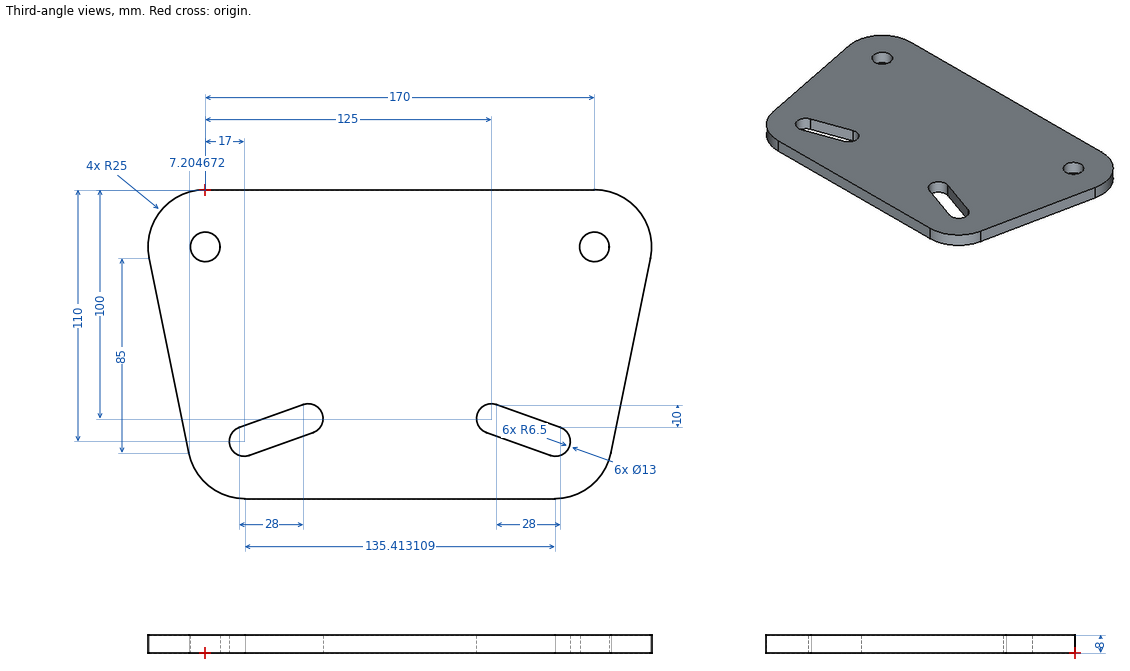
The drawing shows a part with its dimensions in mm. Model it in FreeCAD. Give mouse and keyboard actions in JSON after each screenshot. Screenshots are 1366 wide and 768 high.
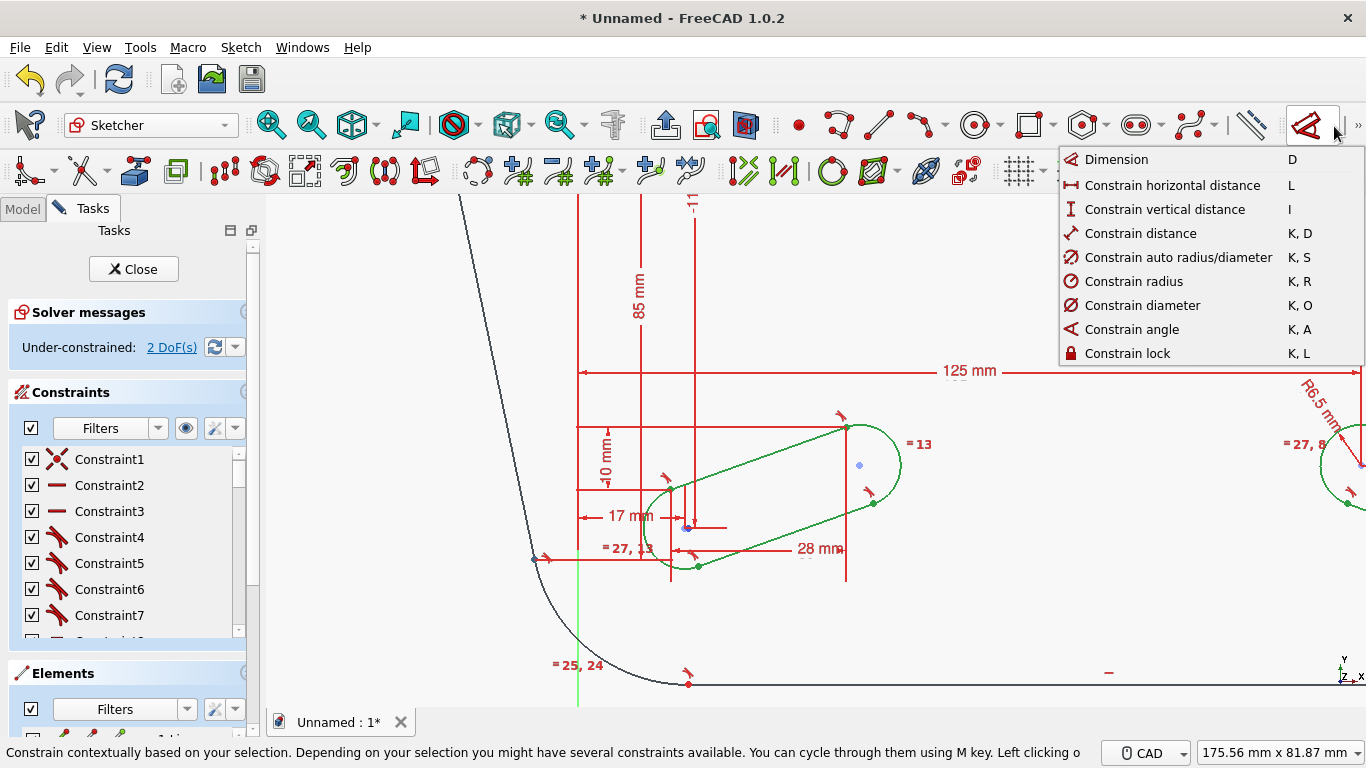
{"action": "left_click", "coordinate": [1212, 185]}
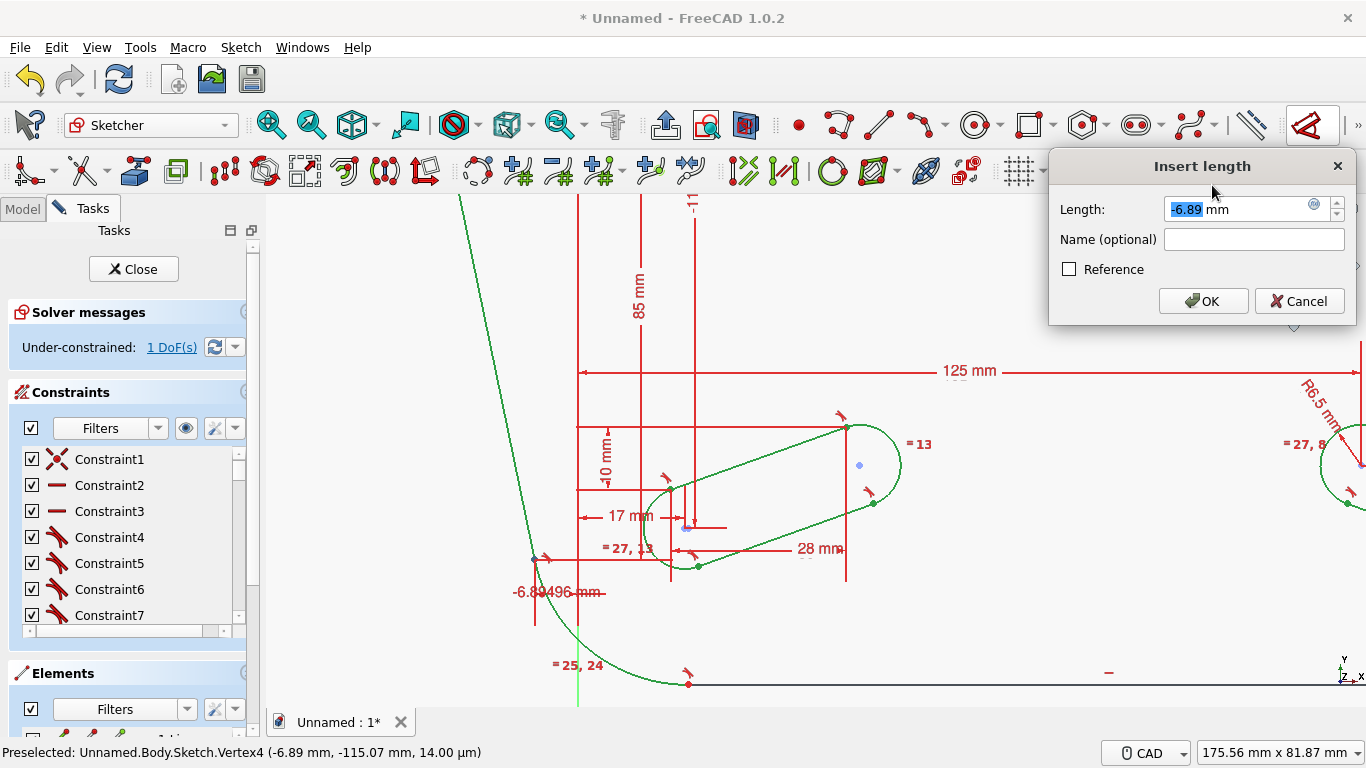
{"action": "type", "text": "-7.204672"}
{"action": "key", "text": "Return"}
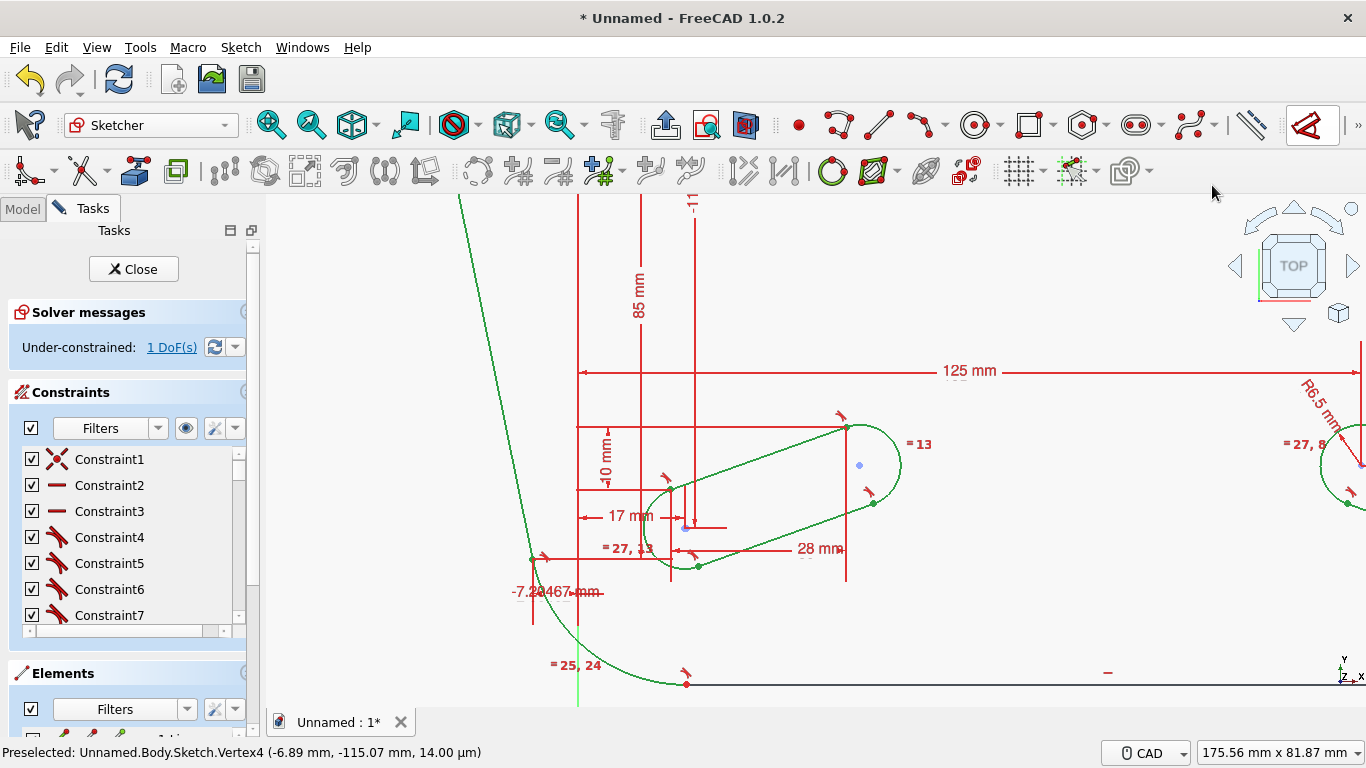
{"action": "scroll", "coordinate": [536, 560], "scroll_direction": "down", "scroll_amount": 5}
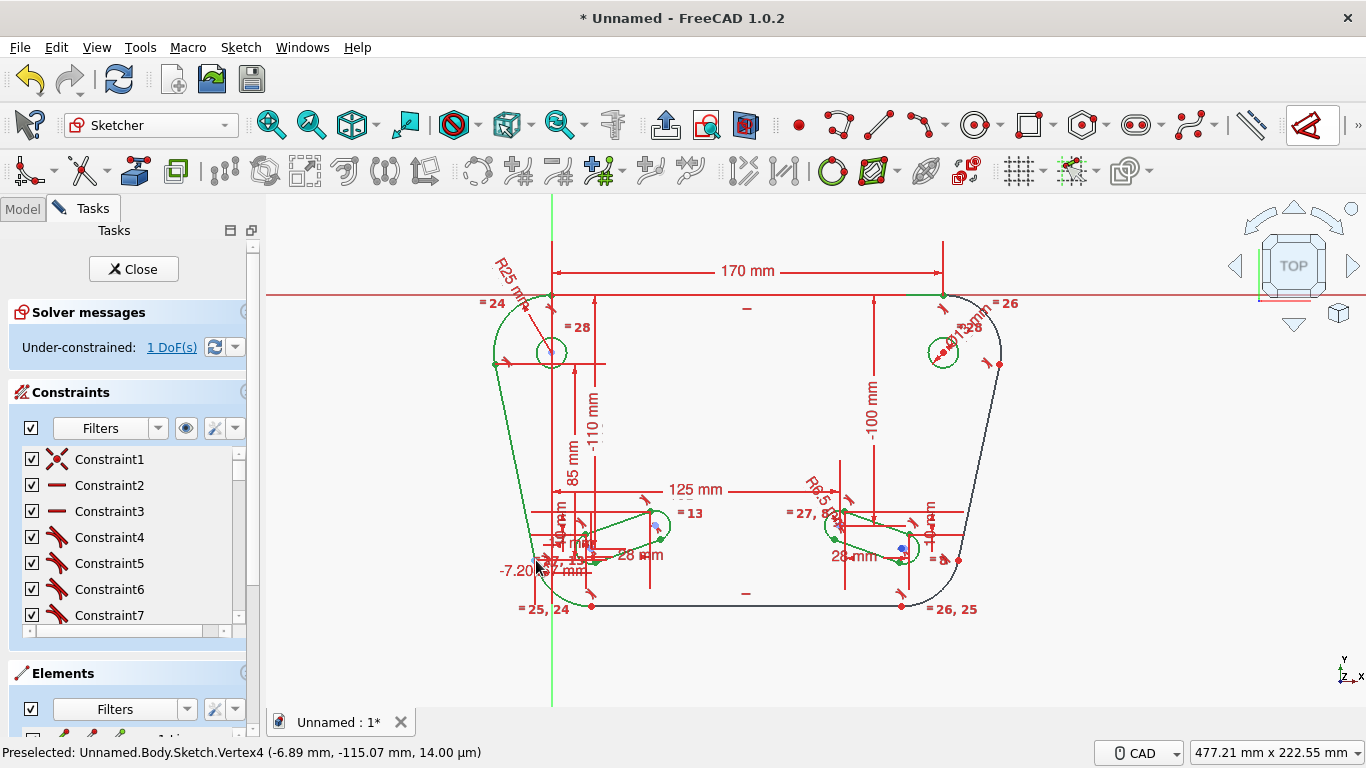
{"action": "left_click", "coordinate": [685, 606]}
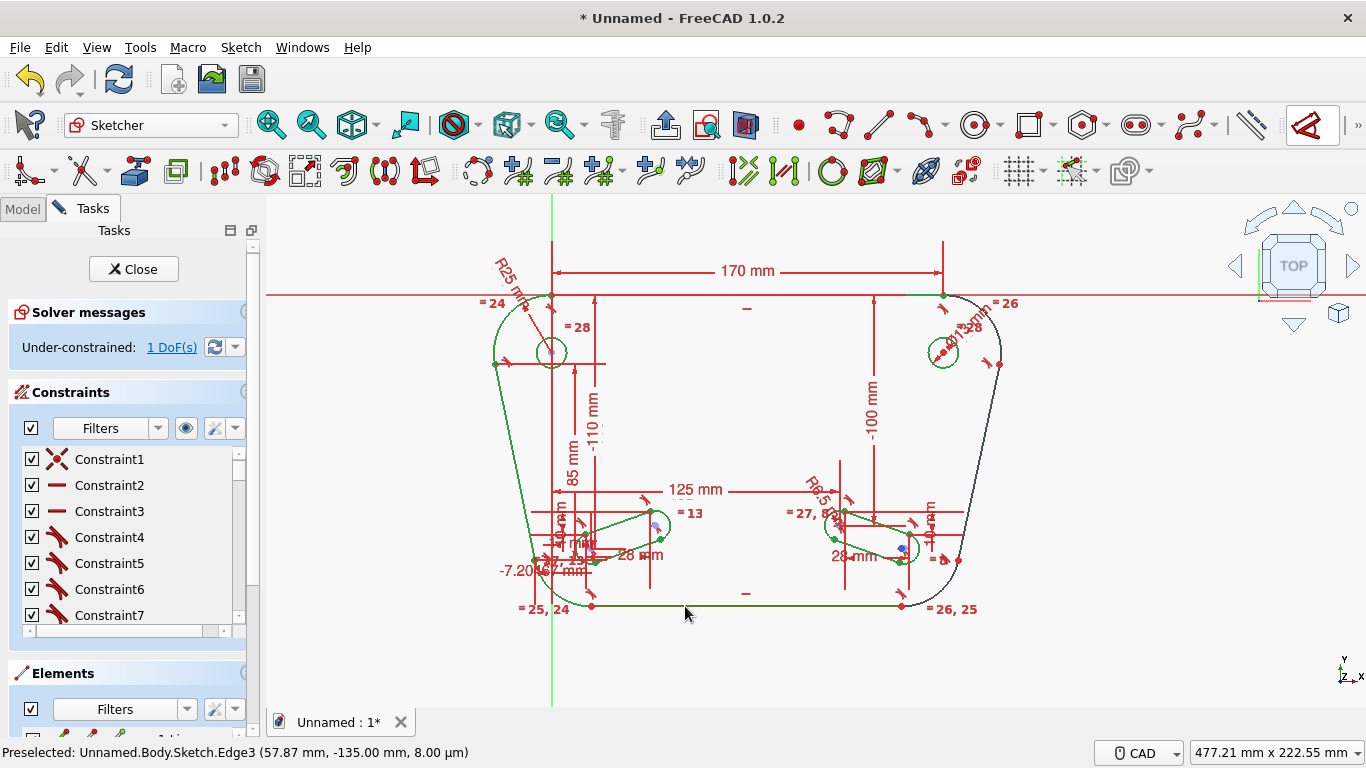
{"action": "key", "text": "l"}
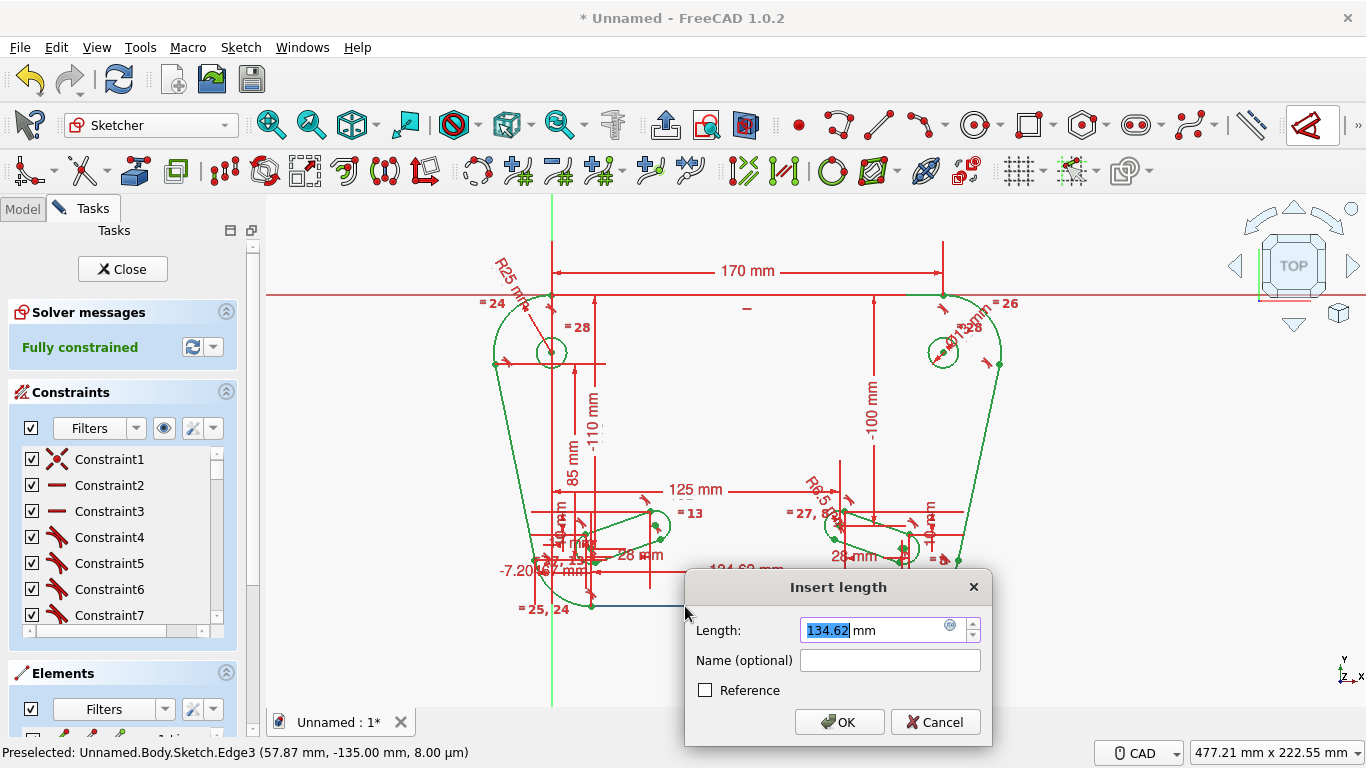
{"action": "type", "text": "135.413109"}
{"action": "key", "text": "Return"}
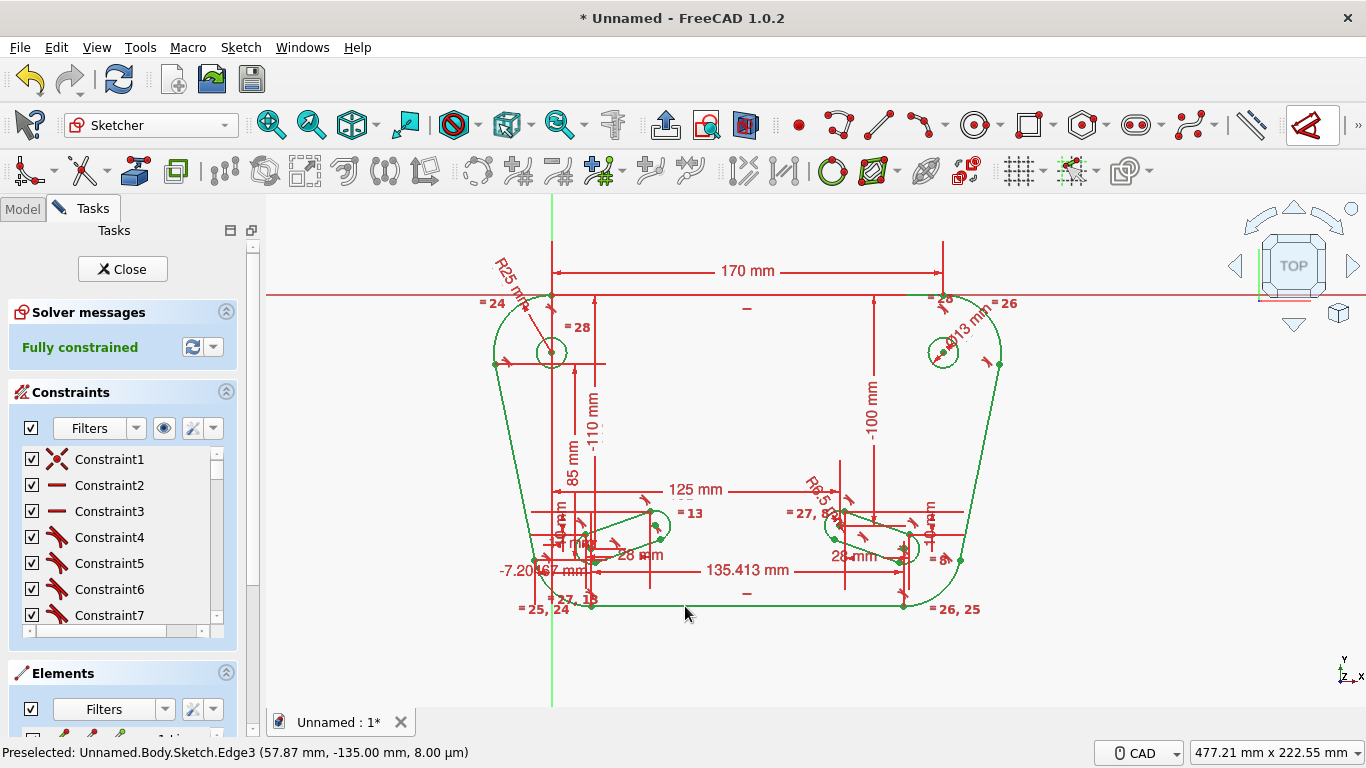
{"action": "left_click", "coordinate": [123, 269]}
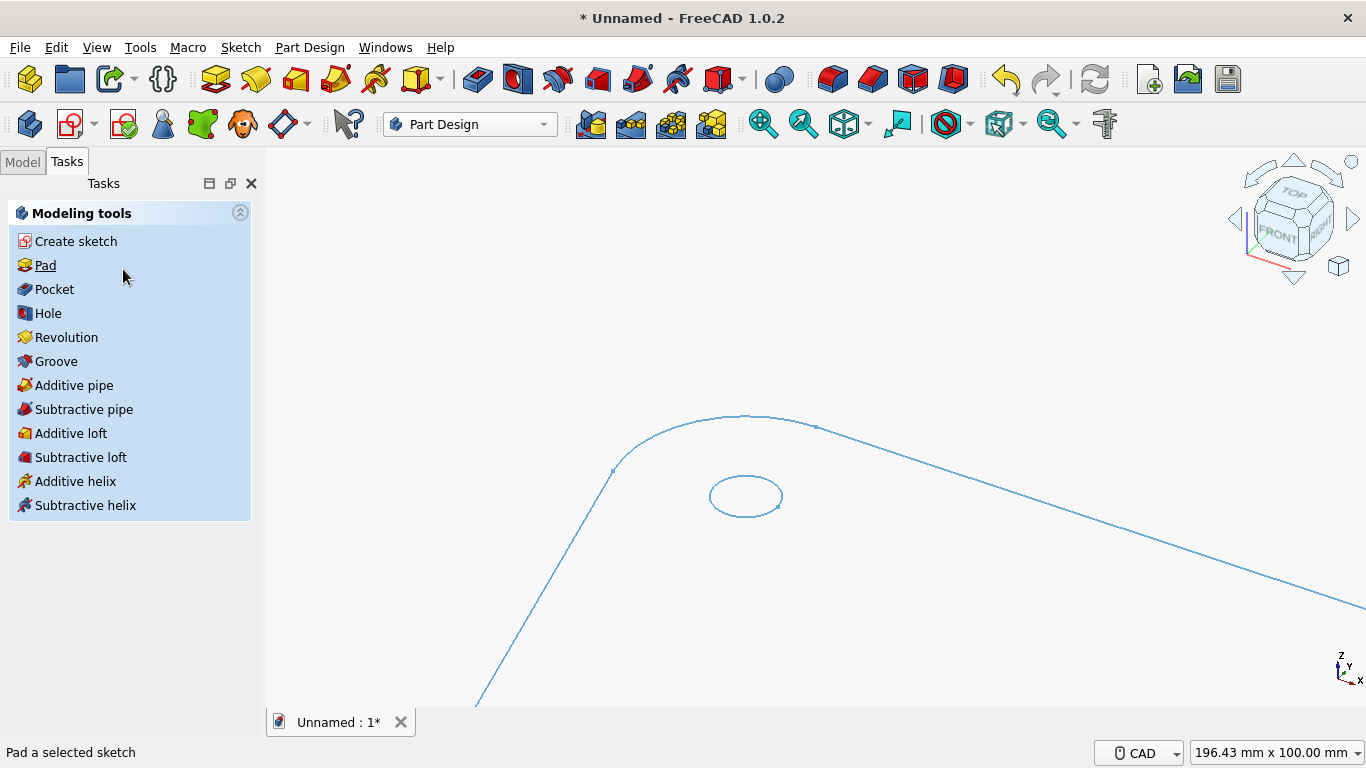
{"action": "left_click", "coordinate": [216, 80]}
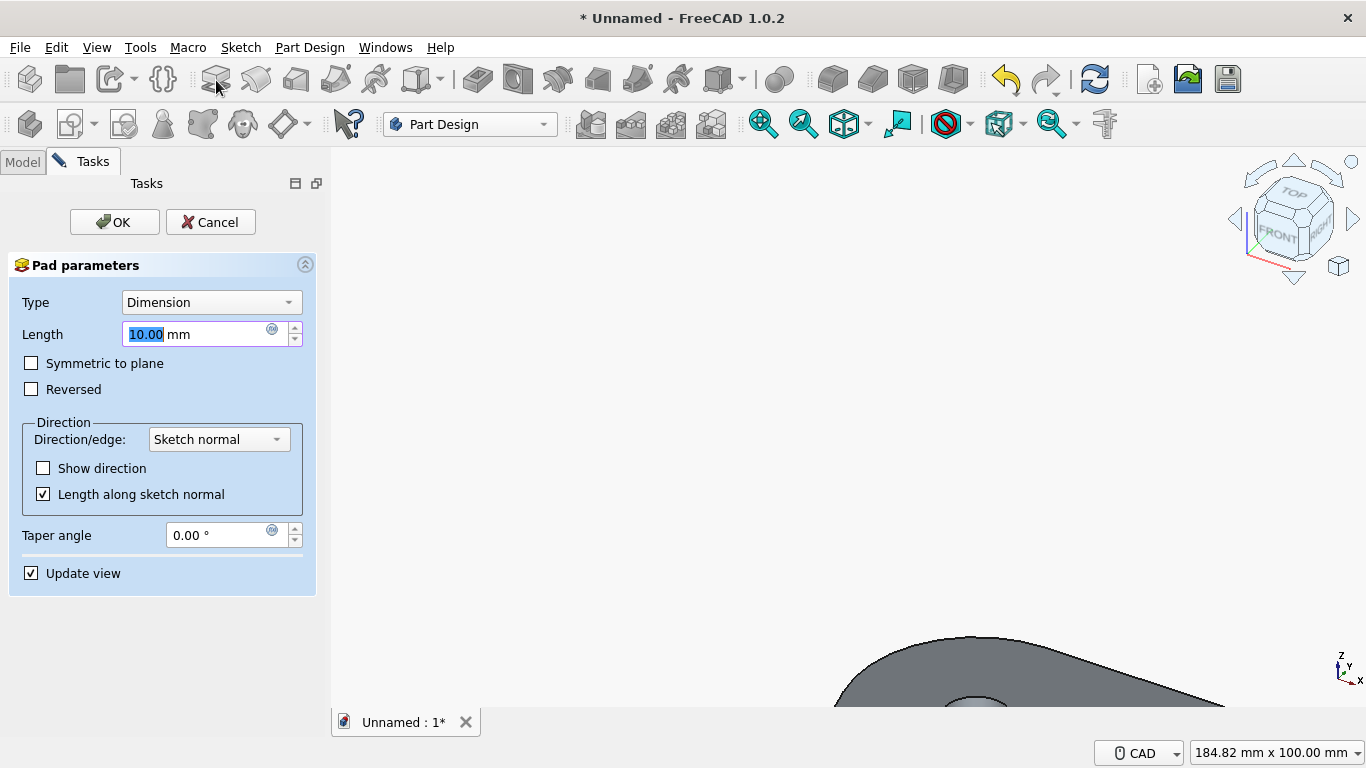
{"action": "type", "text": "8"}
{"action": "key", "text": "Tab"}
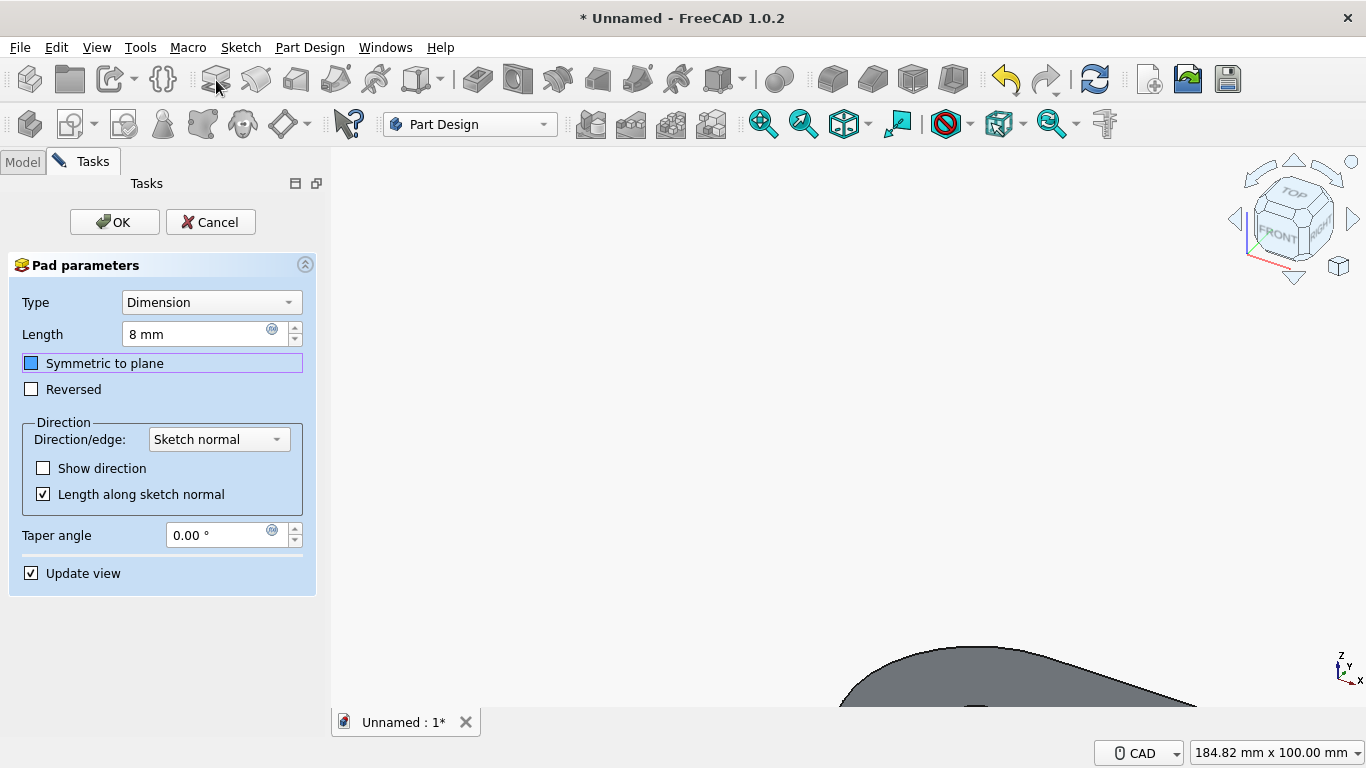
{"action": "left_click", "coordinate": [115, 222]}